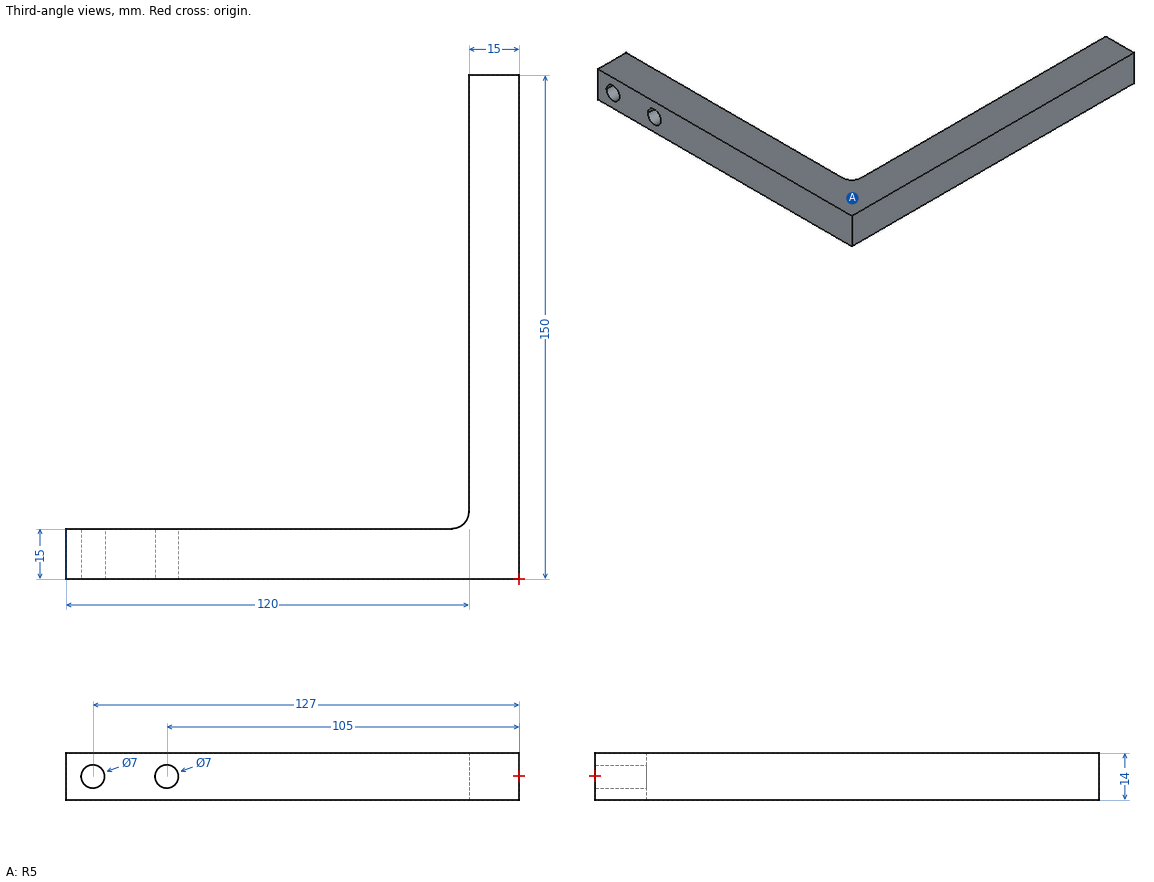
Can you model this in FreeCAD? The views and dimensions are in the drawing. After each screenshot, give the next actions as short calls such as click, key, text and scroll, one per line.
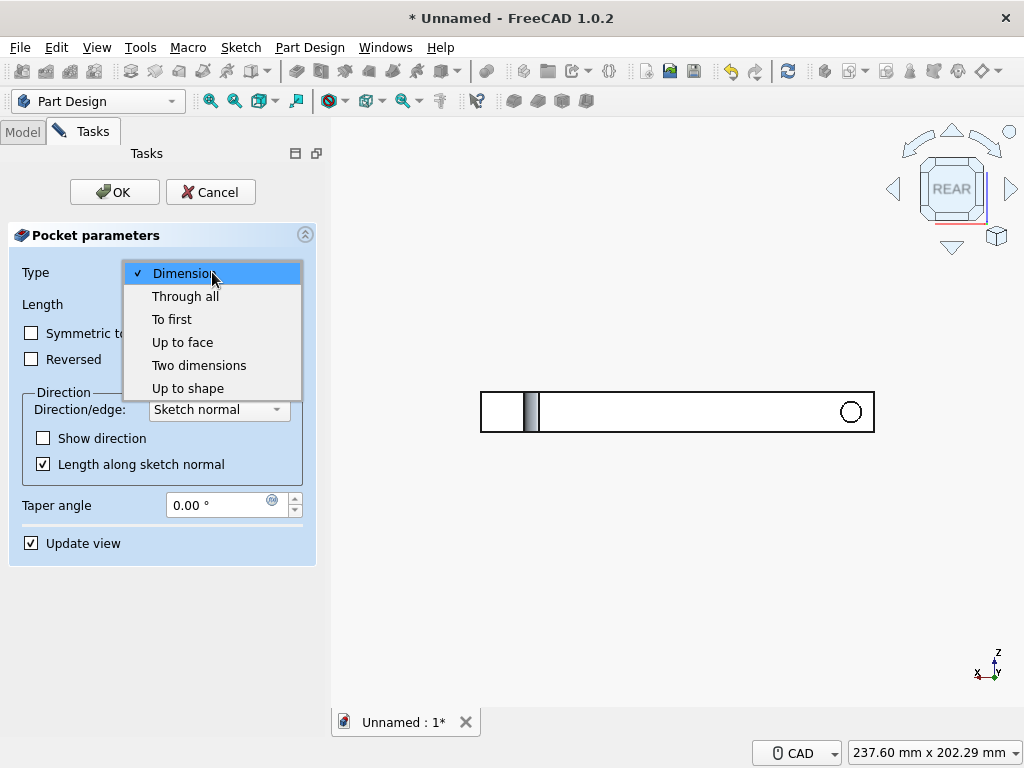
click(212, 320)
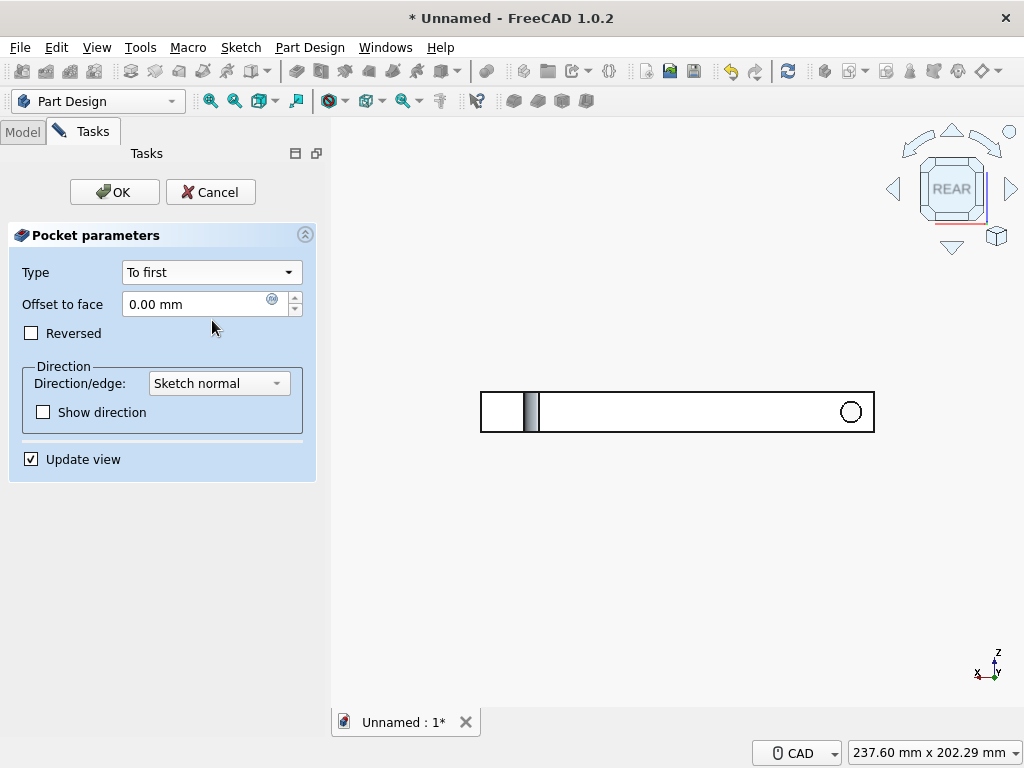
click(115, 192)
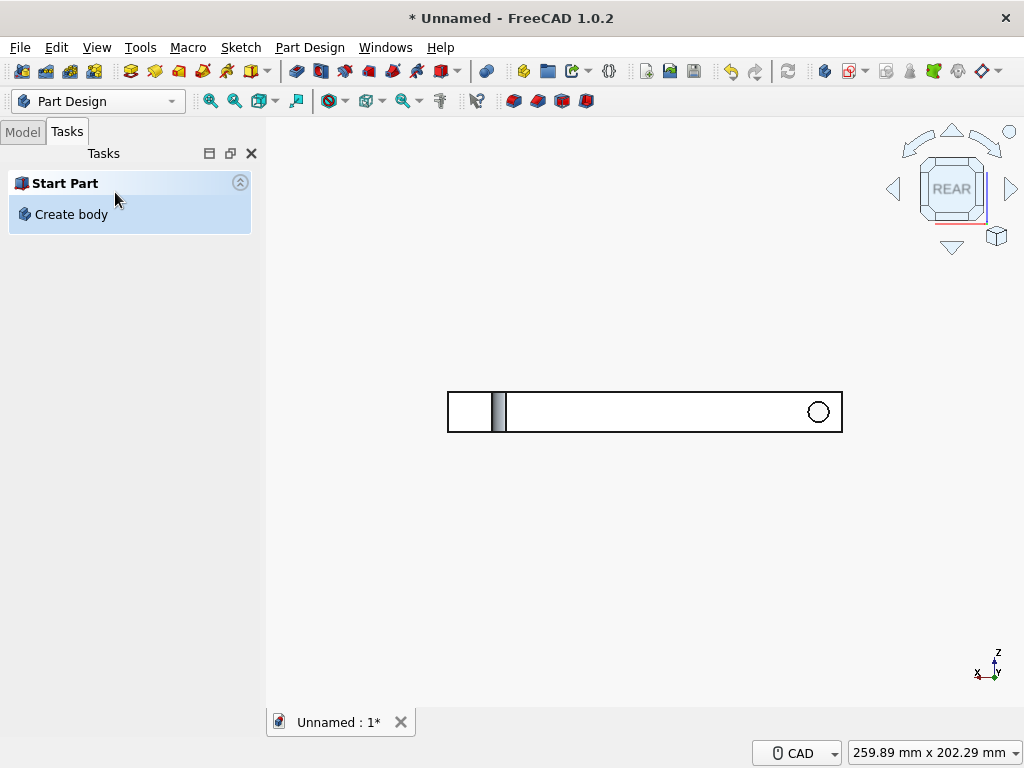
click(530, 411)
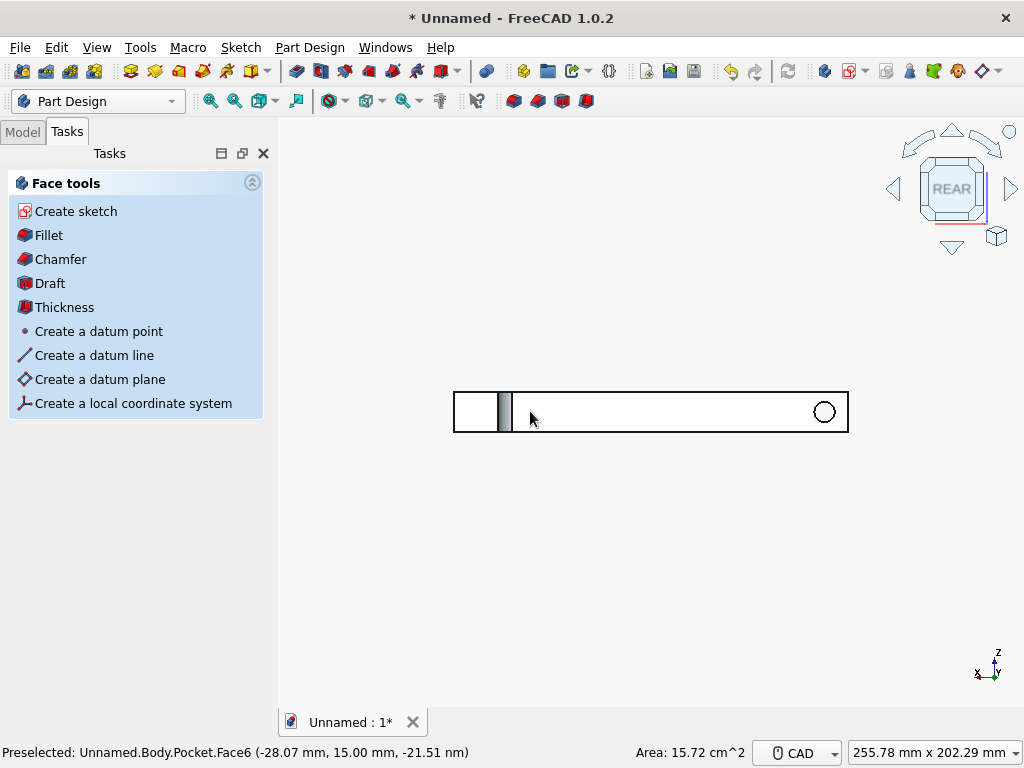
click(850, 72)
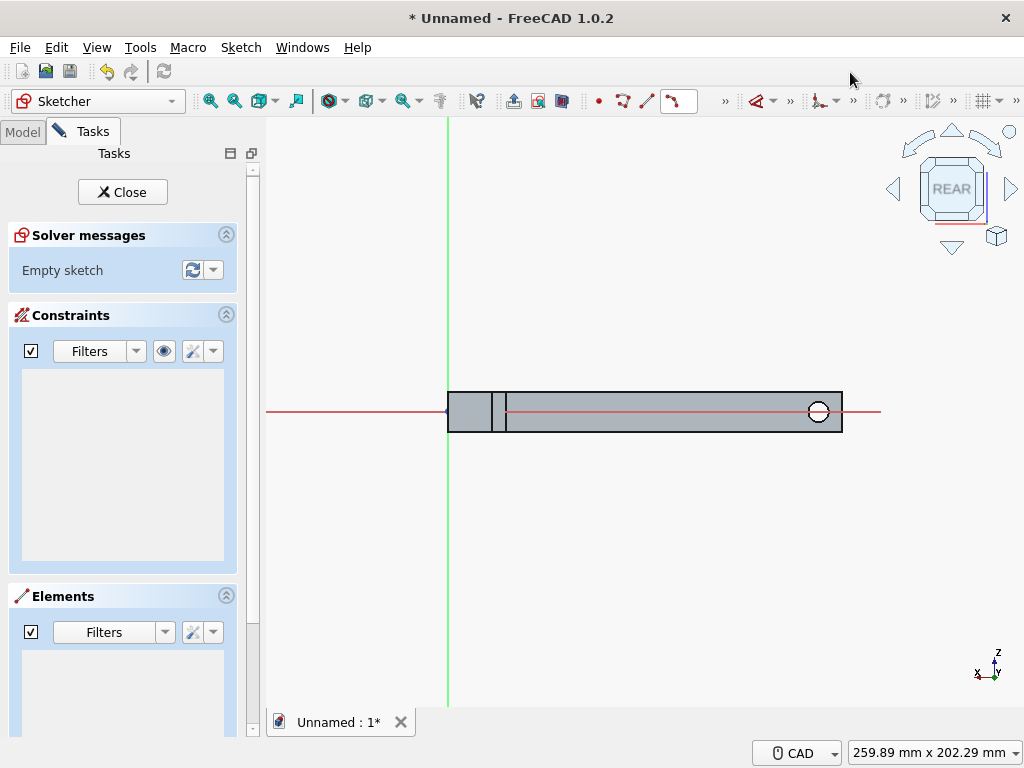
scroll(764, 412, up, 15)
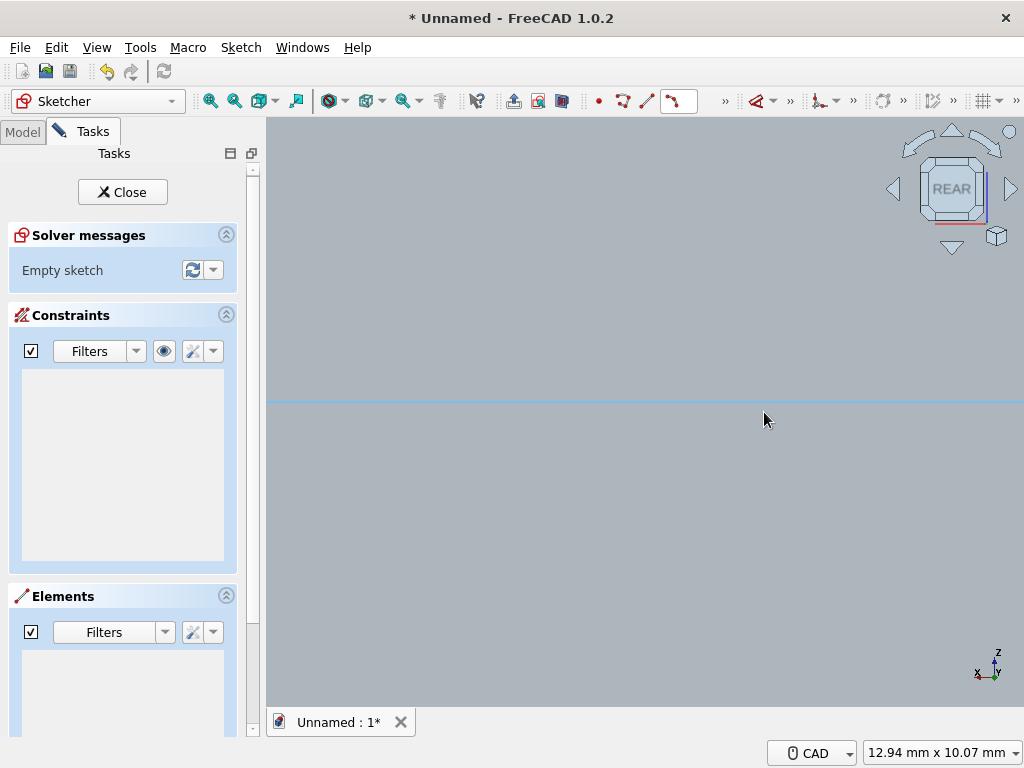
key(g)
key(c)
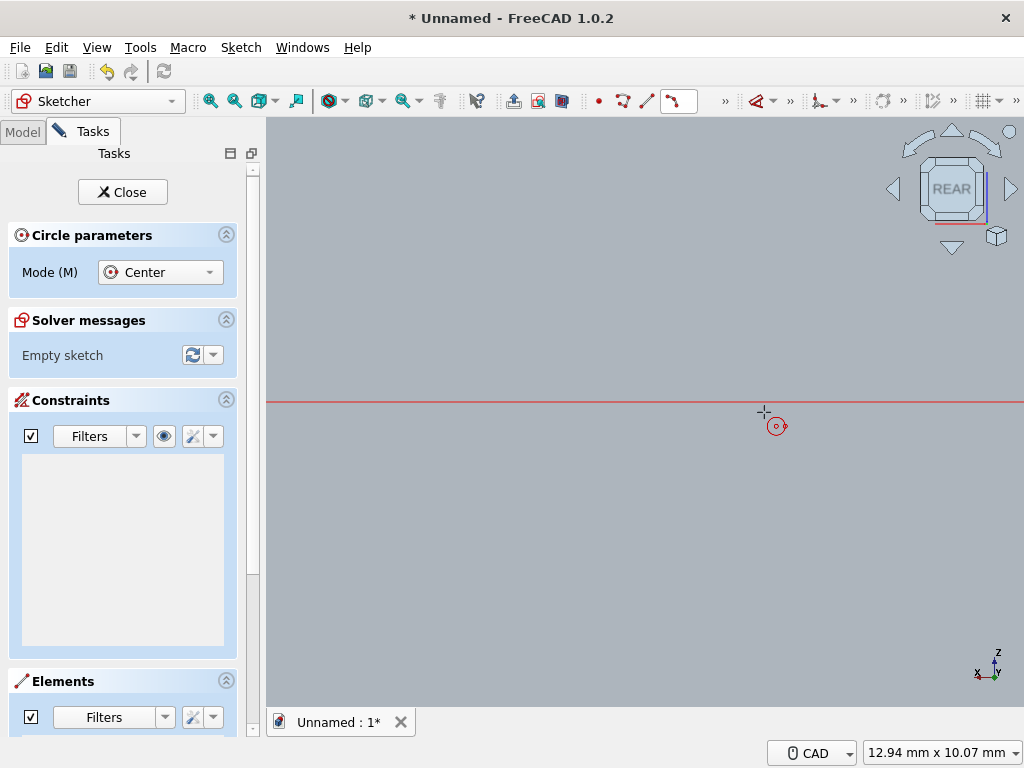
click(558, 402)
click(703, 257)
key(Escape)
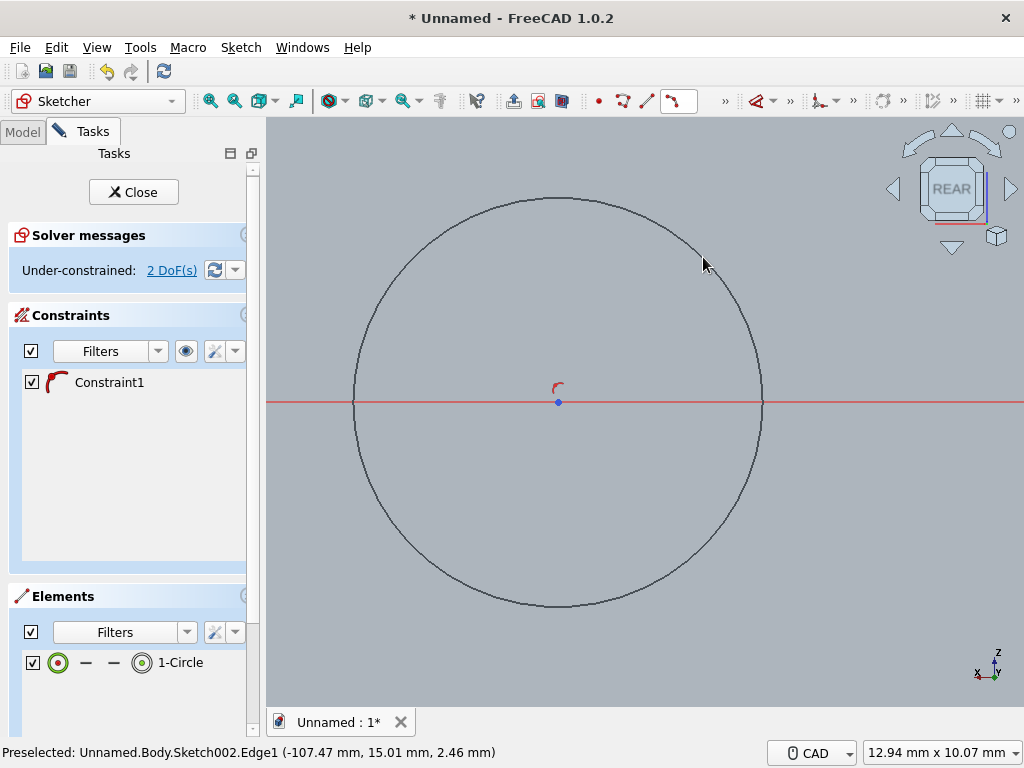
click(756, 102)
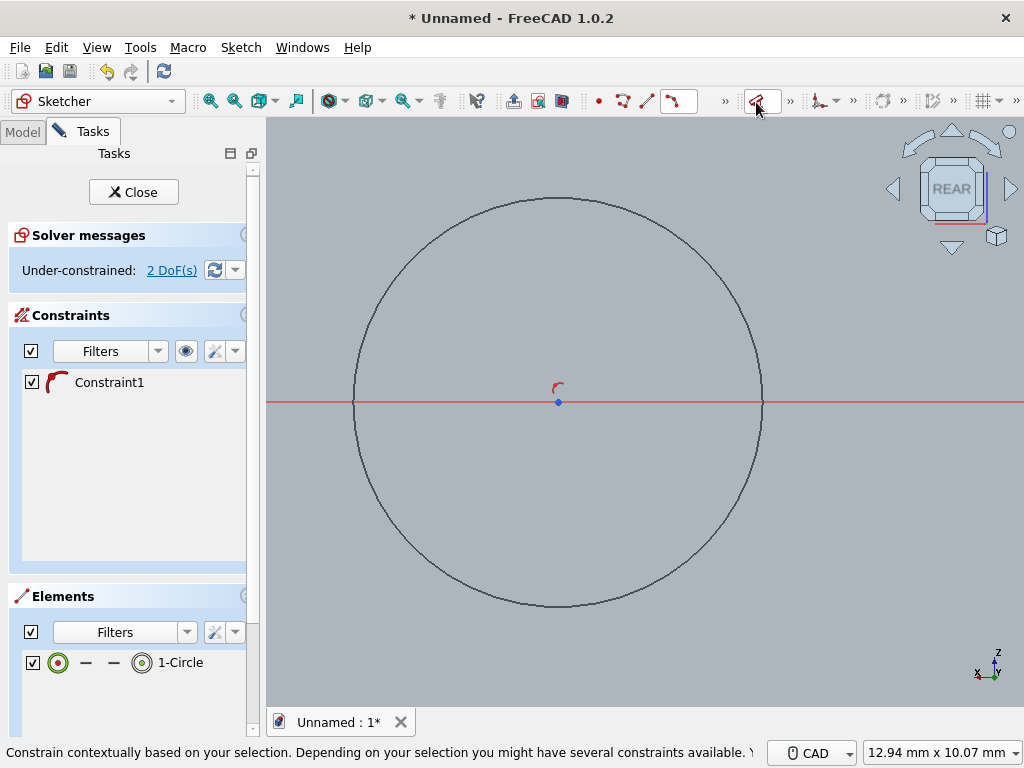
click(702, 257)
click(725, 234)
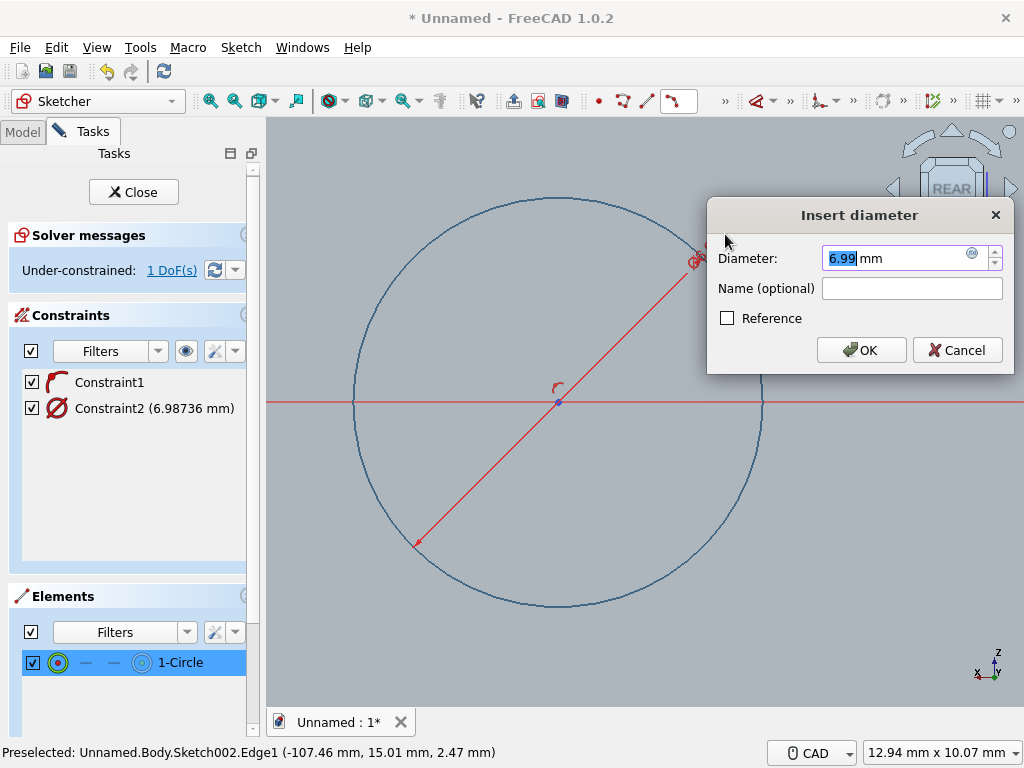
text(7)
key(Return)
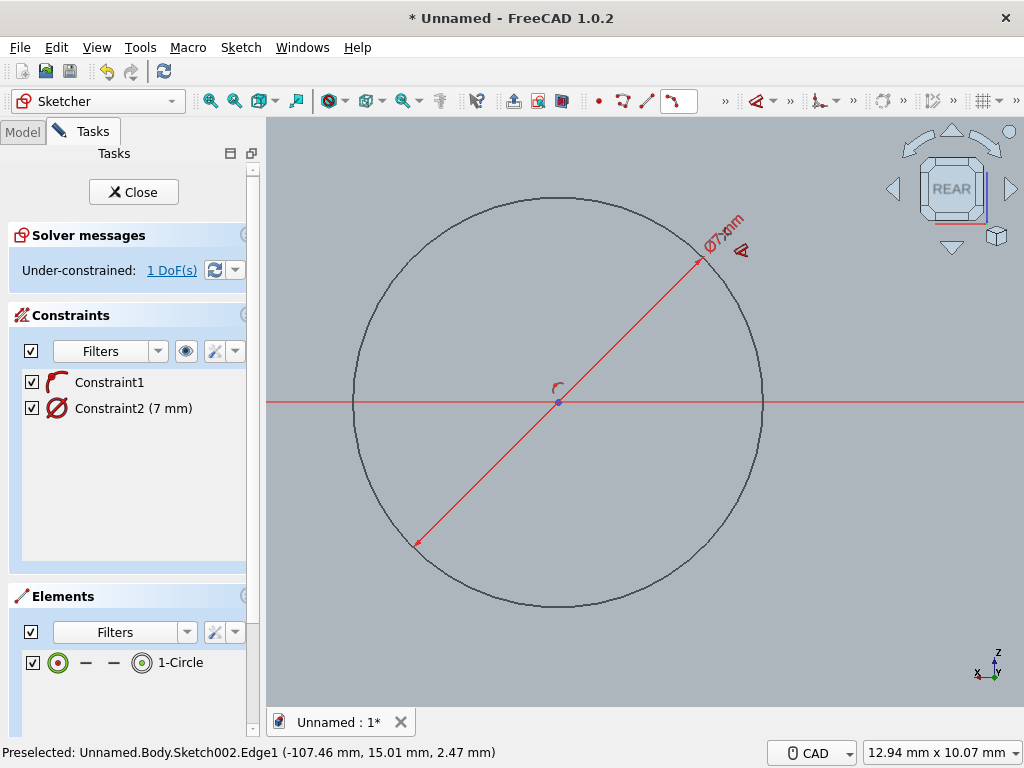
click(558, 402)
click(426, 436)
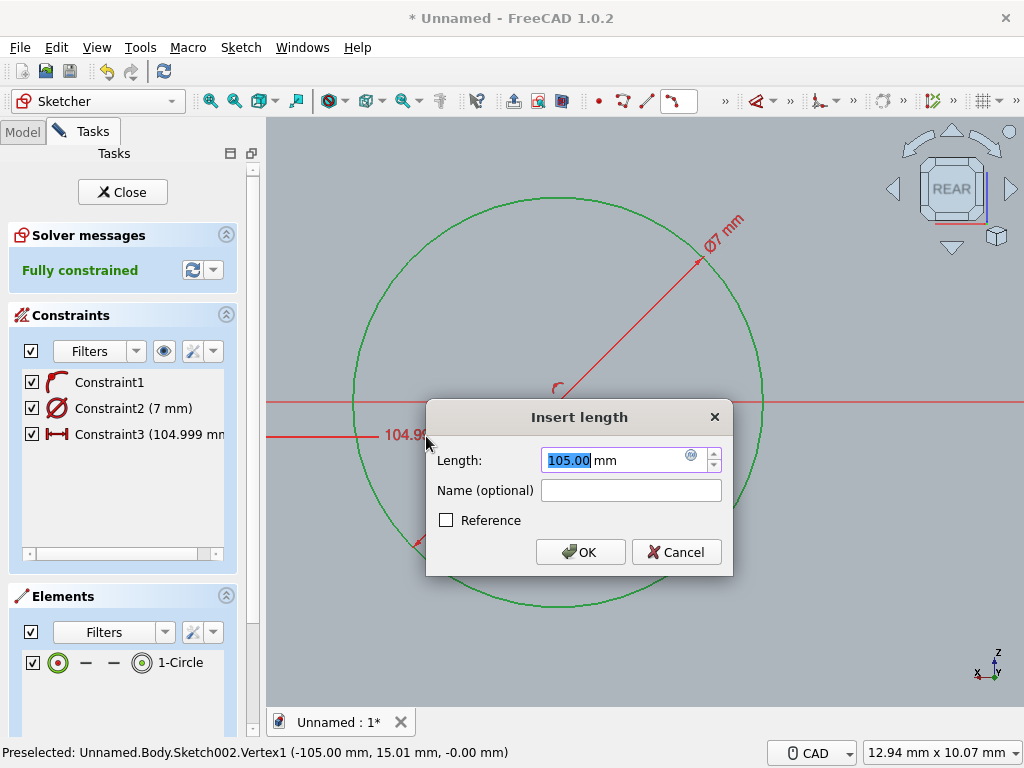
text(105)
key(Return)
key(Escape)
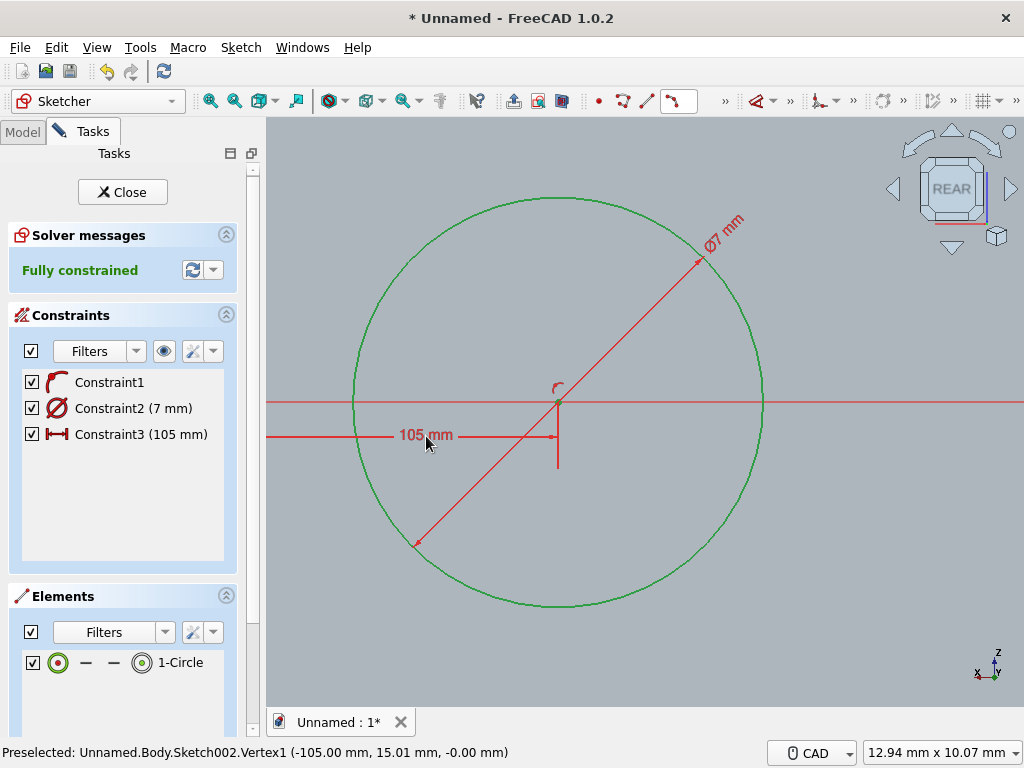
click(123, 192)